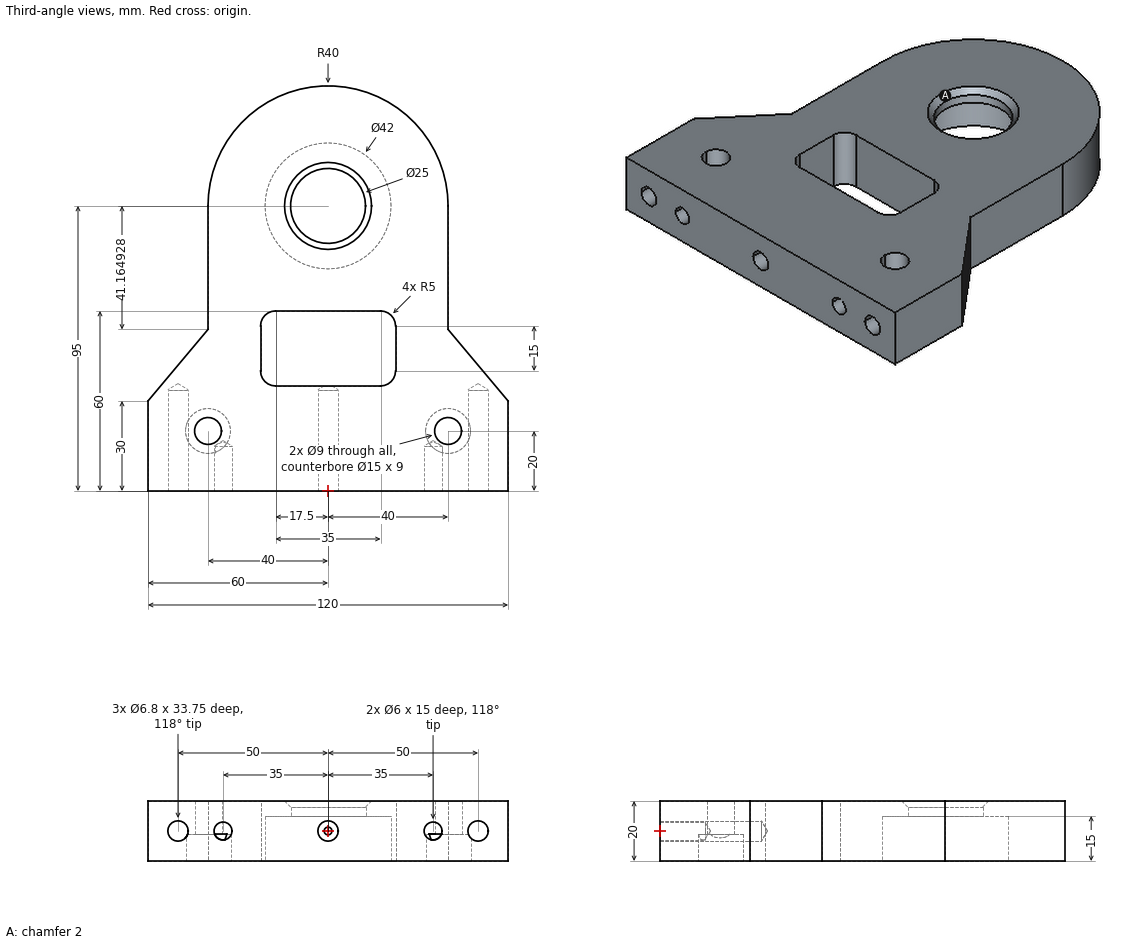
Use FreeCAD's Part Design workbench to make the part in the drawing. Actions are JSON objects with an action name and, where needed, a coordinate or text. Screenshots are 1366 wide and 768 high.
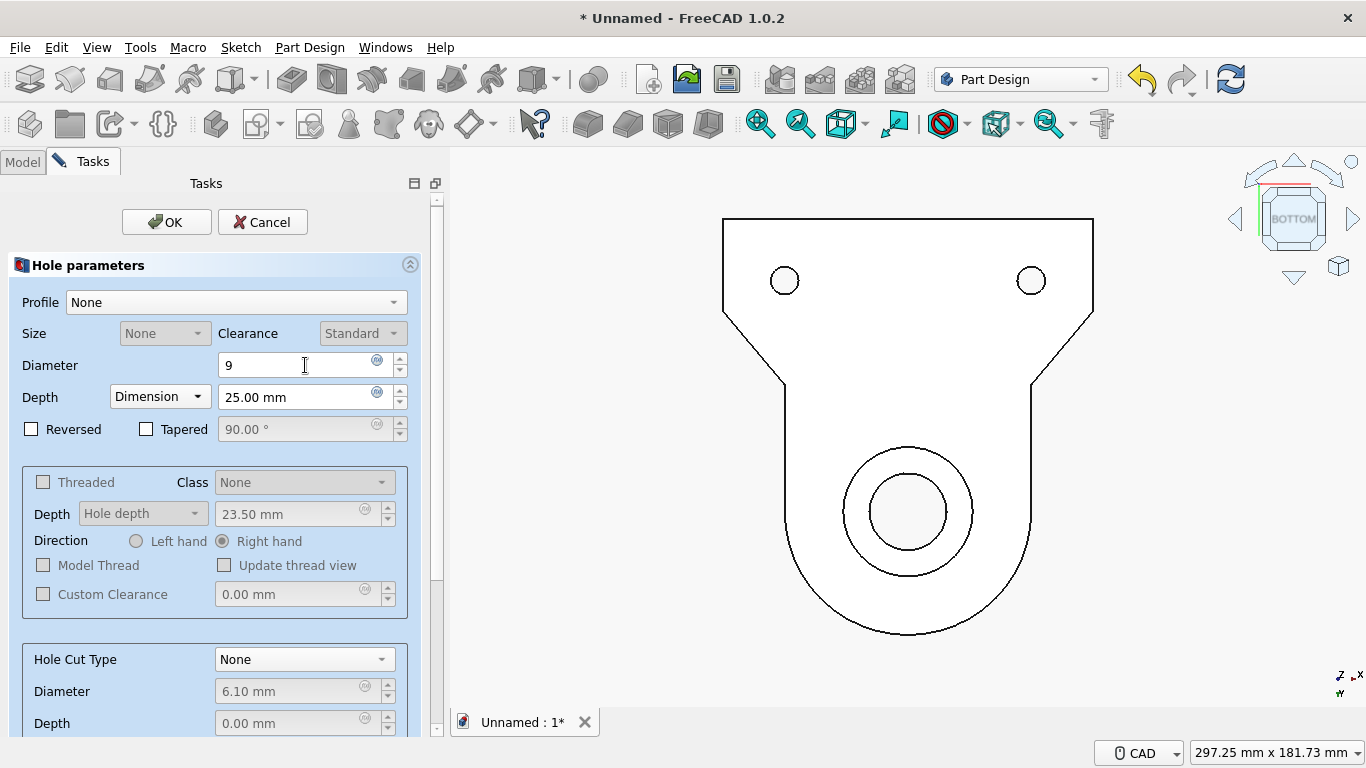
{"action": "left_click", "coordinate": [161, 396]}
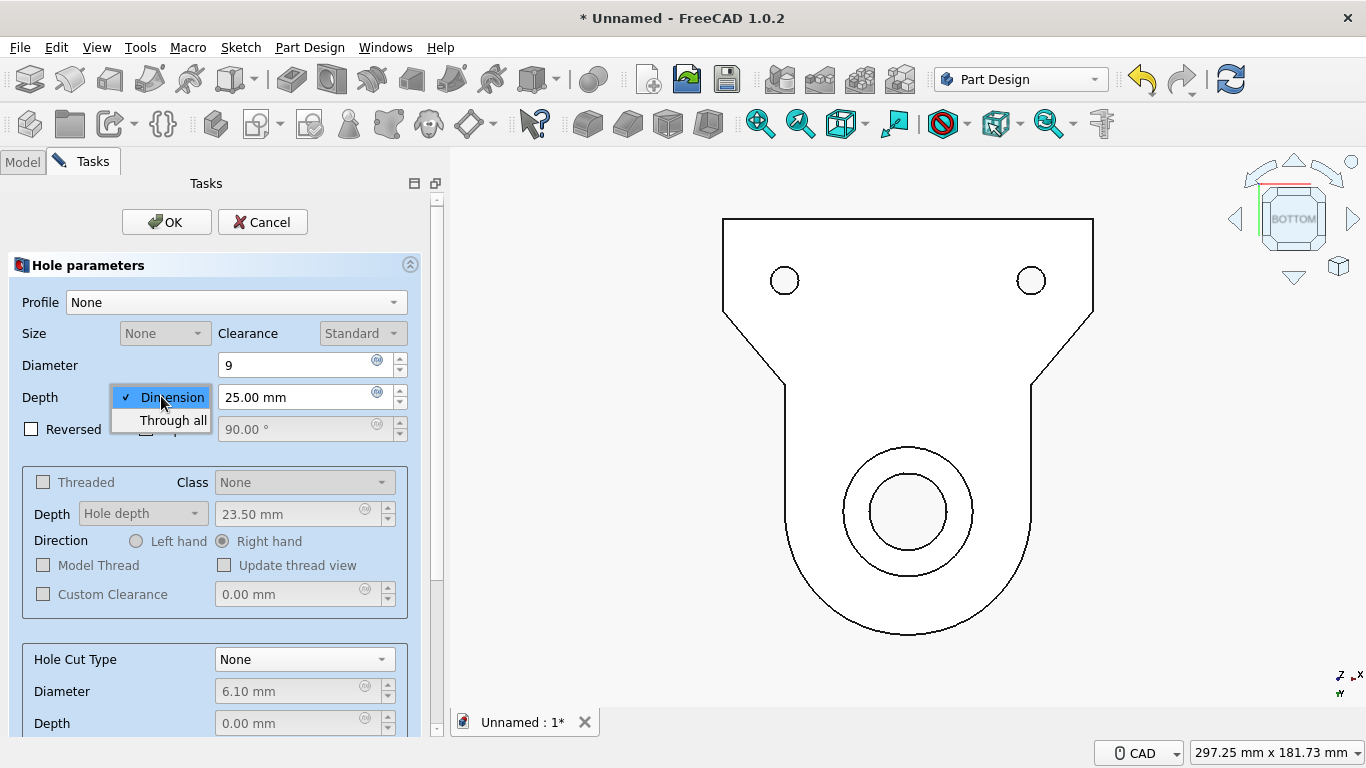
{"action": "left_click", "coordinate": [160, 420]}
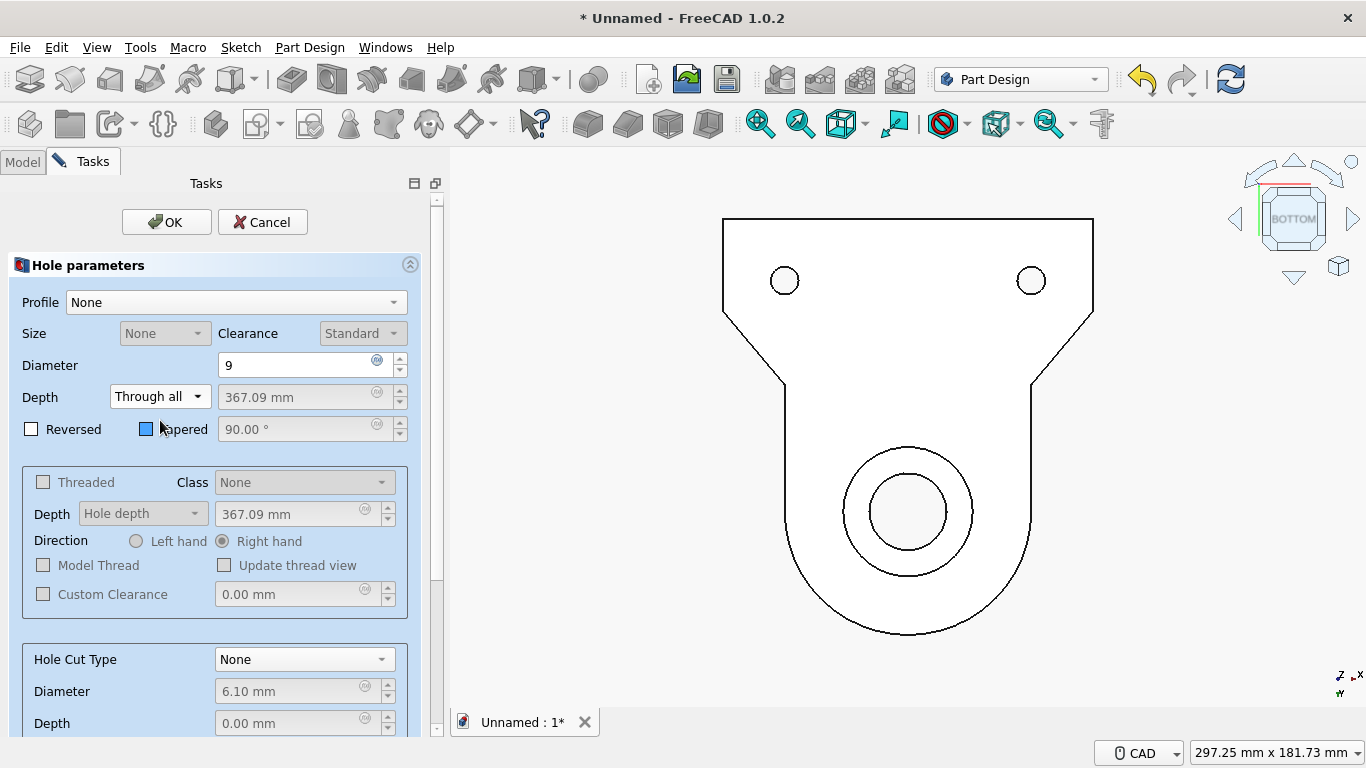
{"action": "left_click", "coordinate": [306, 660]}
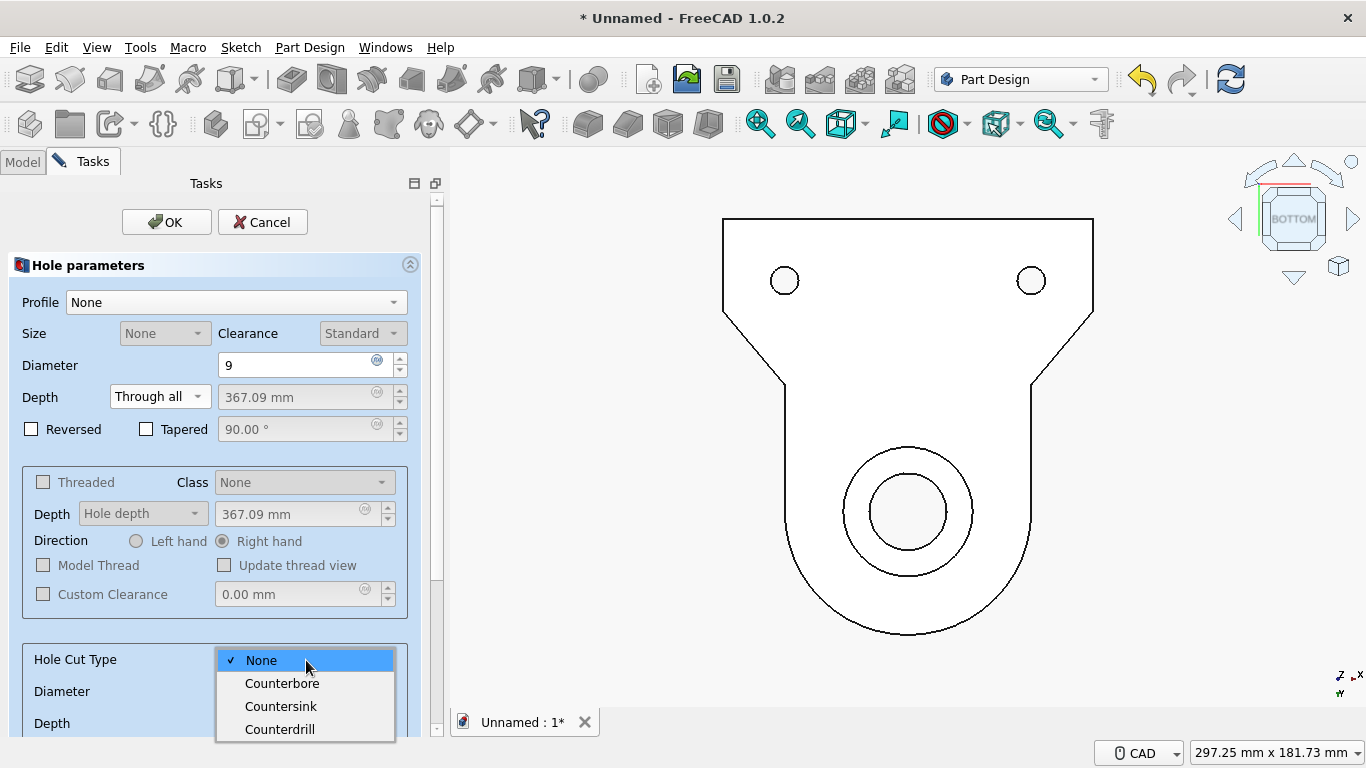
{"action": "left_click", "coordinate": [304, 684]}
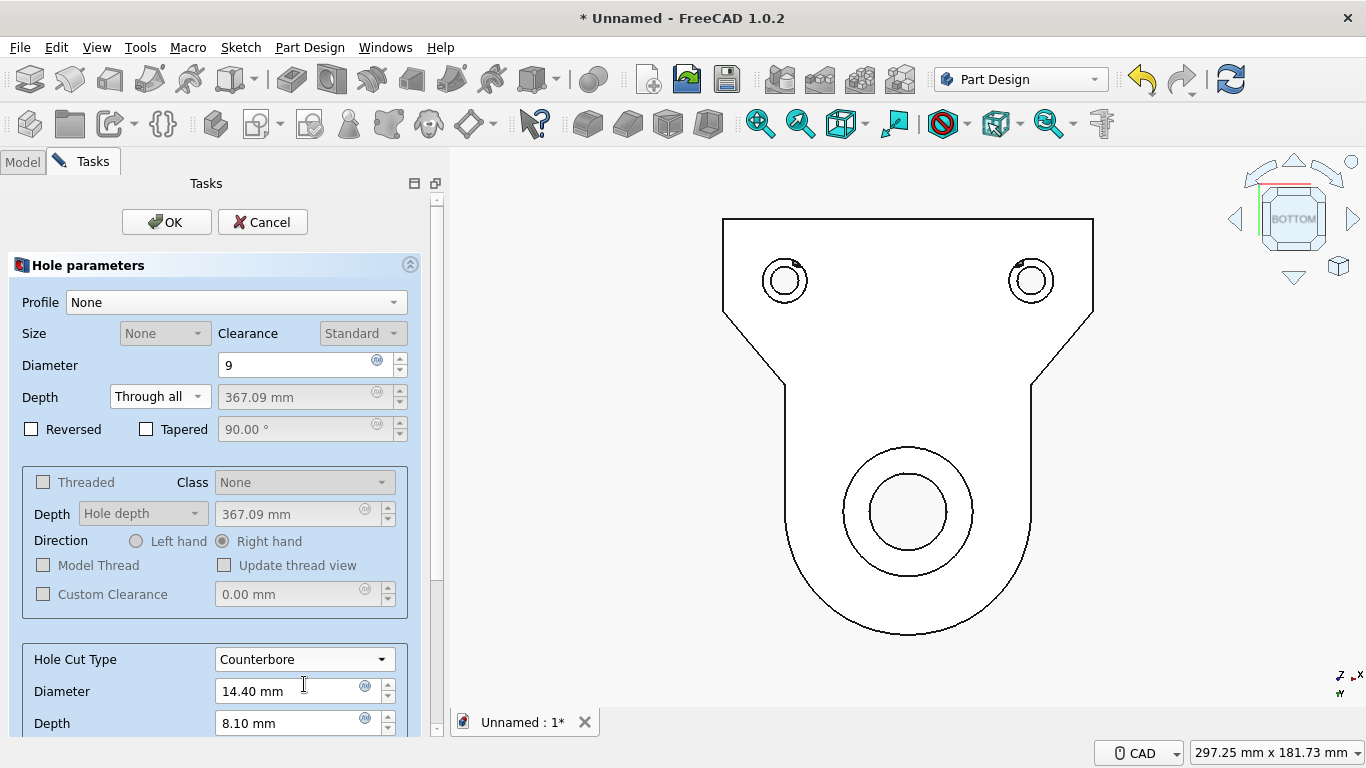
{"action": "triple_click", "coordinate": [298, 691]}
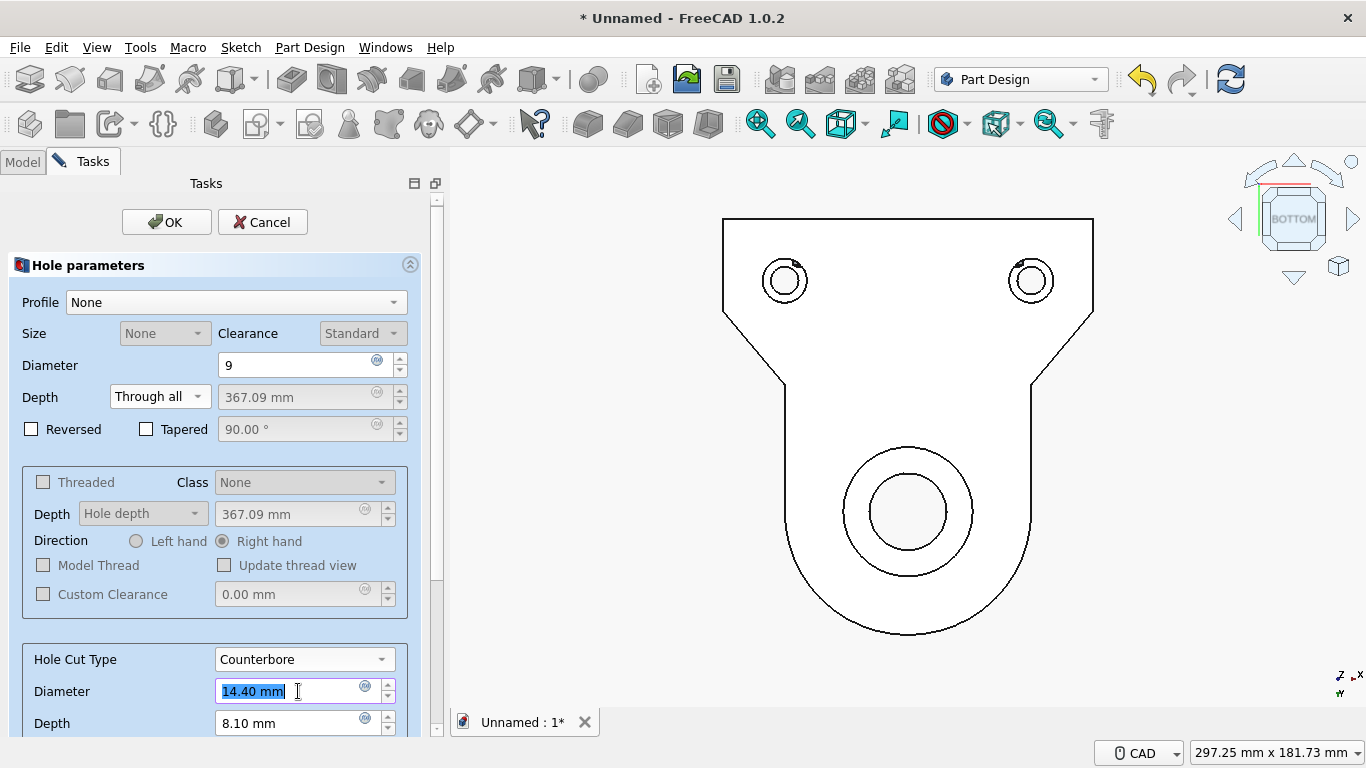
{"action": "type", "text": "15"}
{"action": "key", "text": "Tab"}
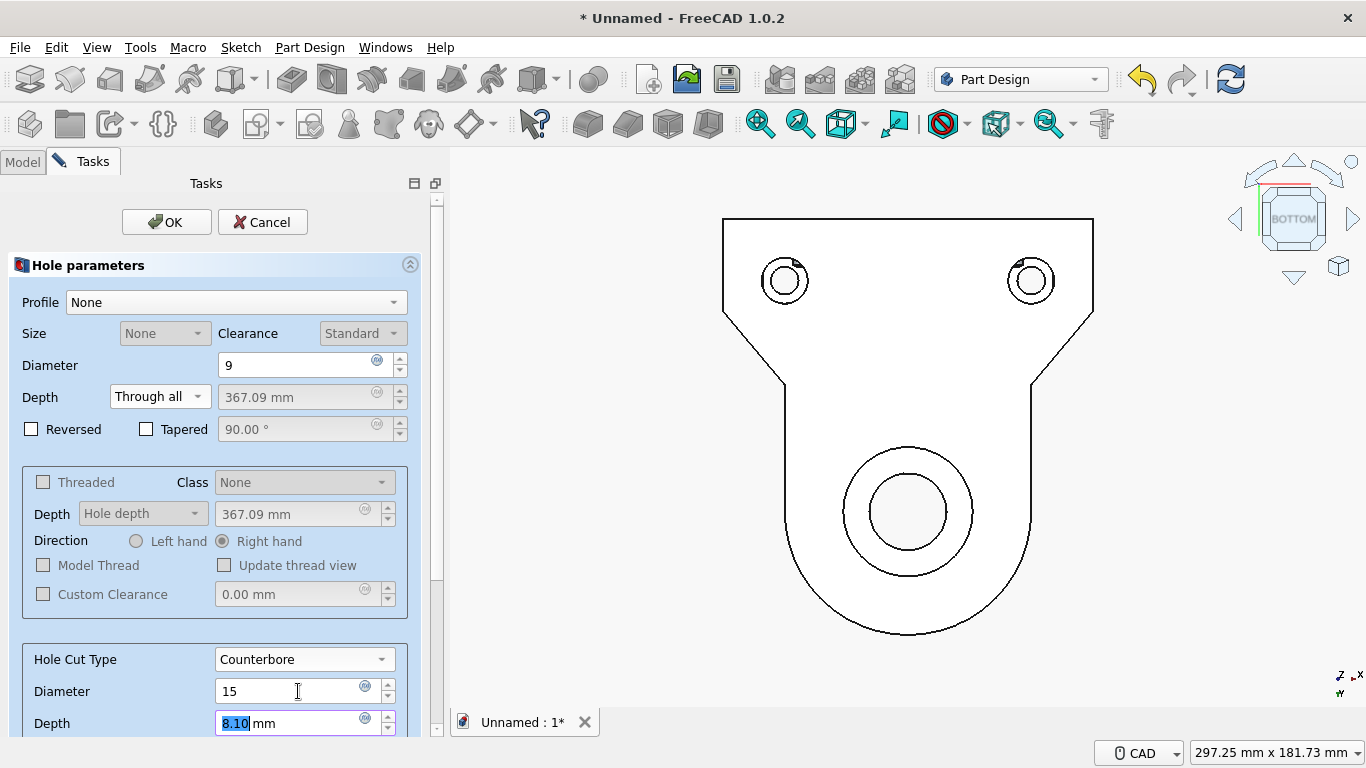
{"action": "type", "text": "9"}
{"action": "key", "text": "Tab"}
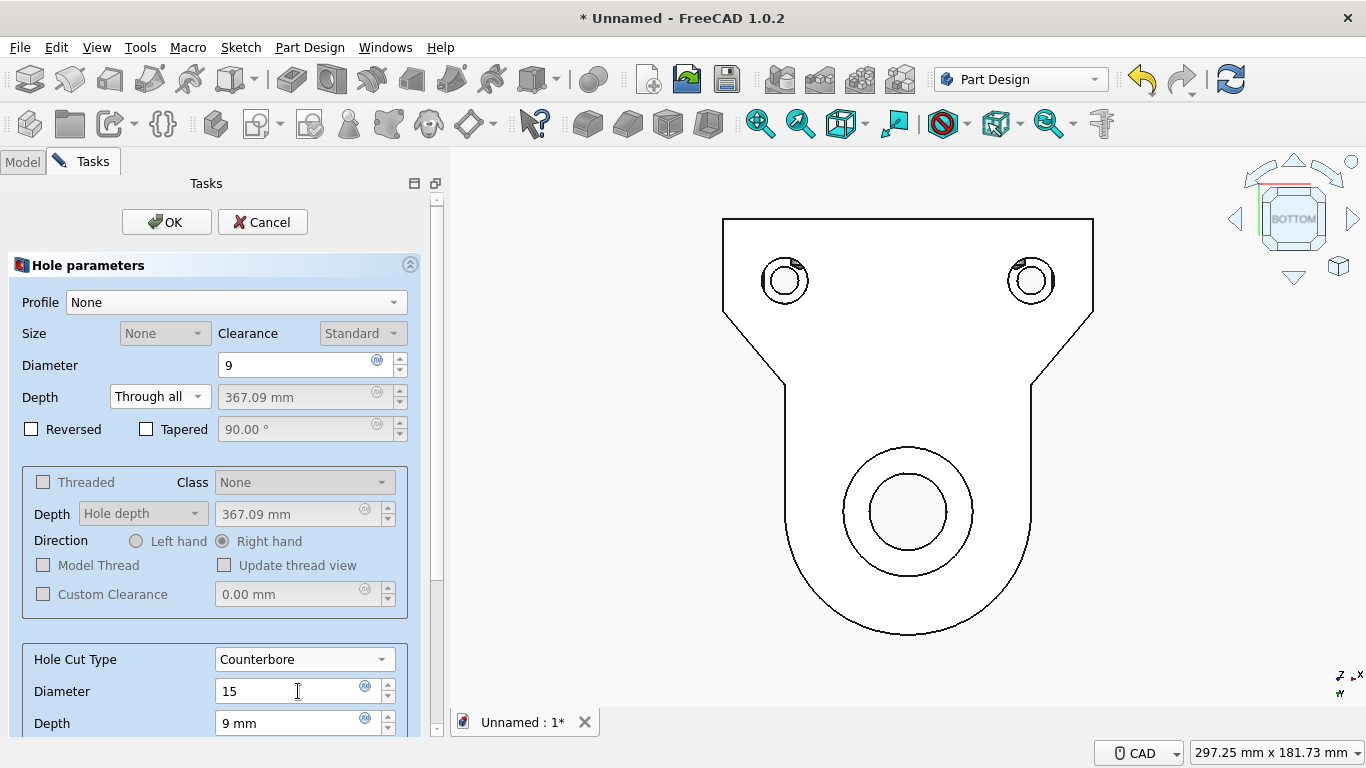
{"action": "left_click", "coordinate": [167, 222]}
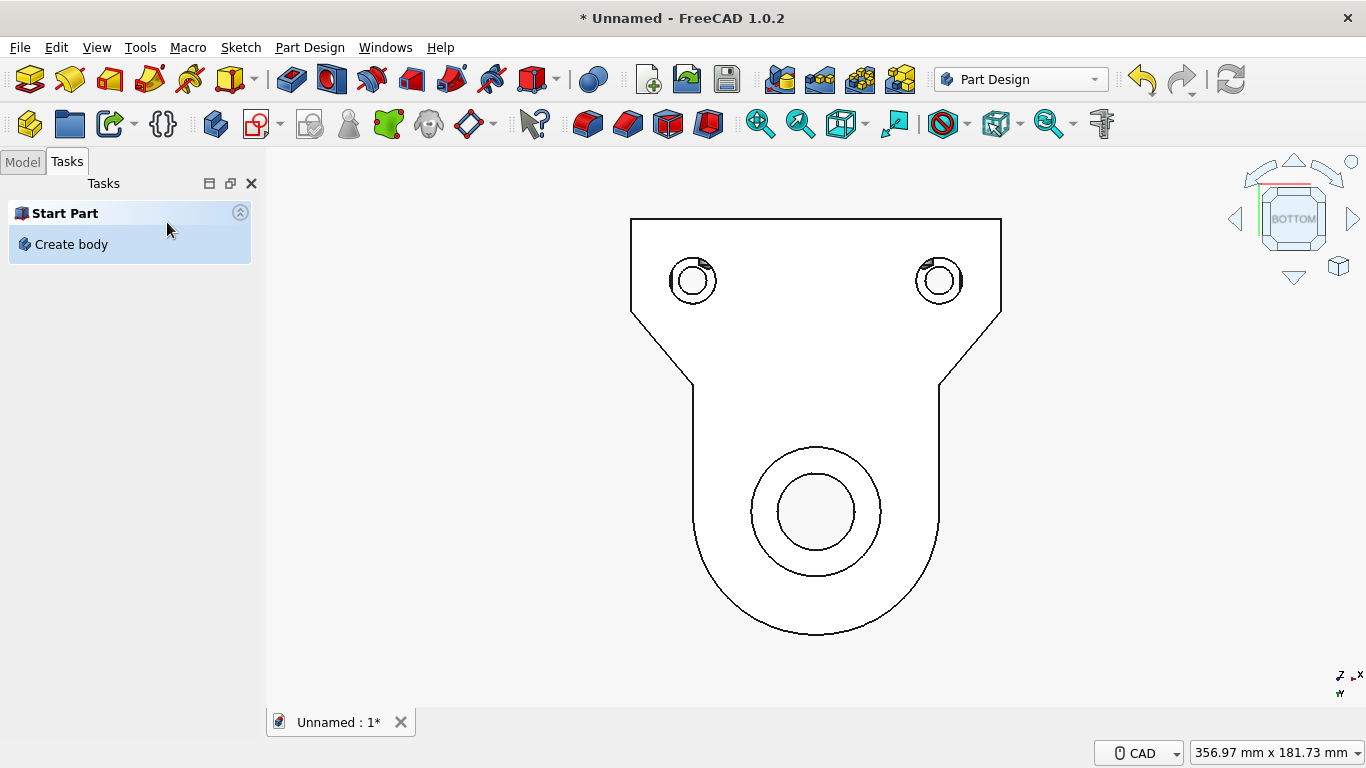
{"action": "left_click", "coordinate": [816, 307]}